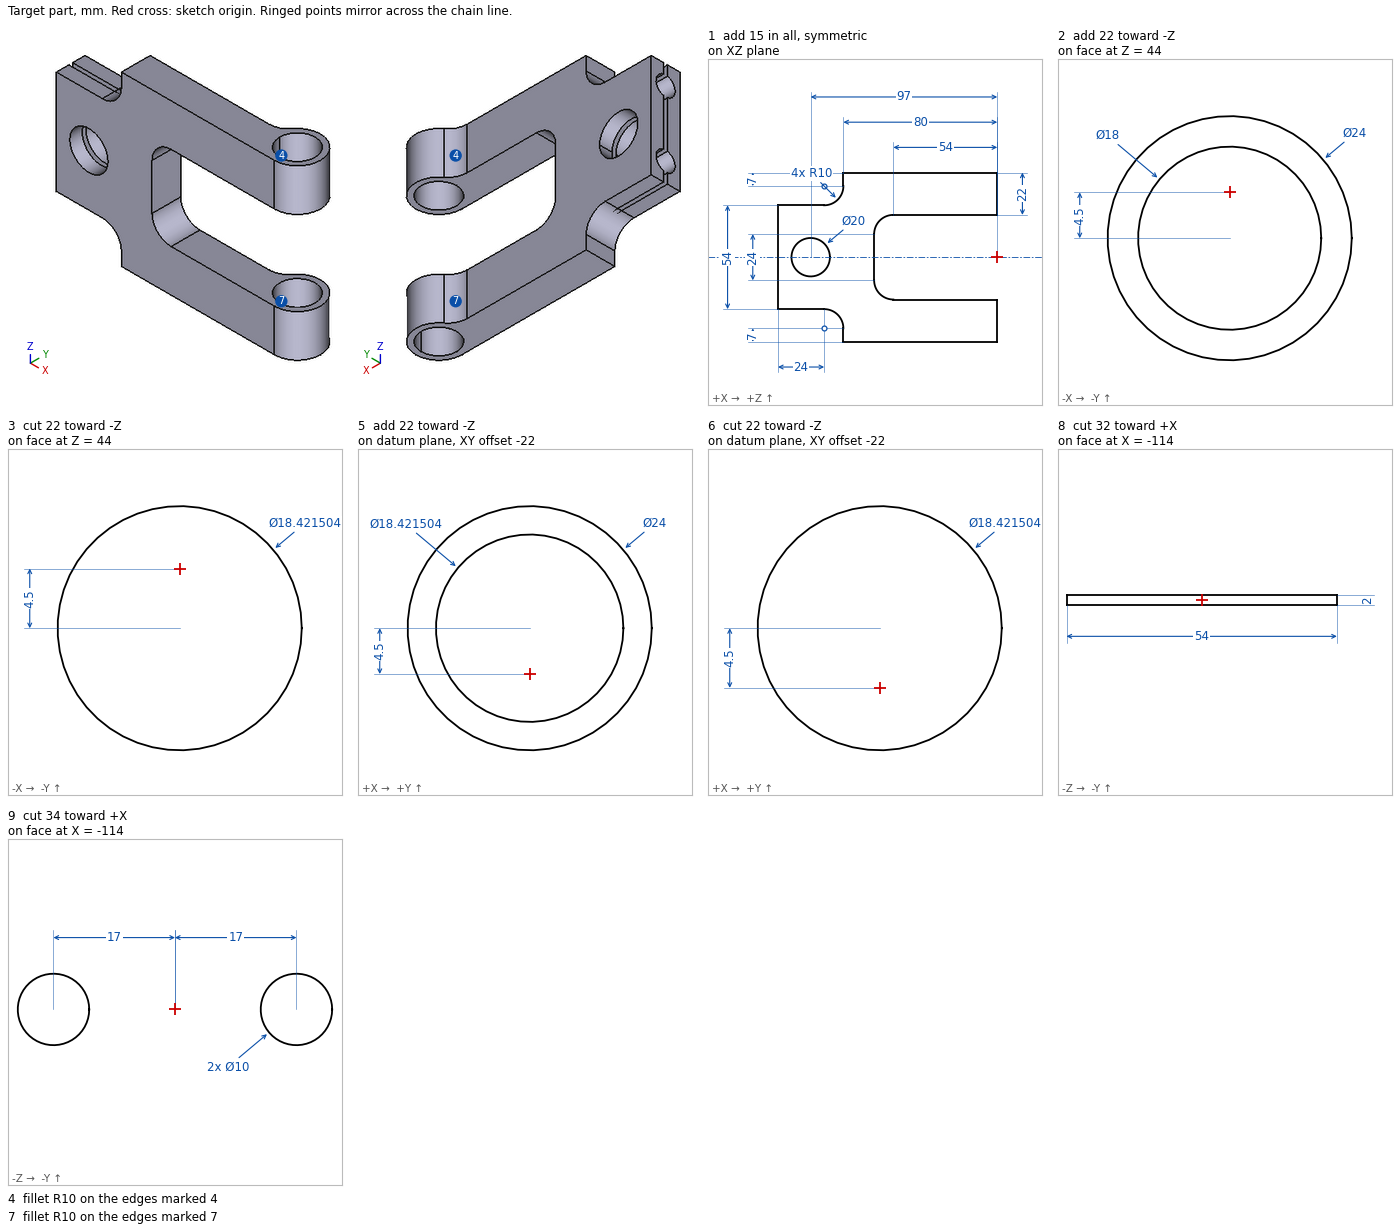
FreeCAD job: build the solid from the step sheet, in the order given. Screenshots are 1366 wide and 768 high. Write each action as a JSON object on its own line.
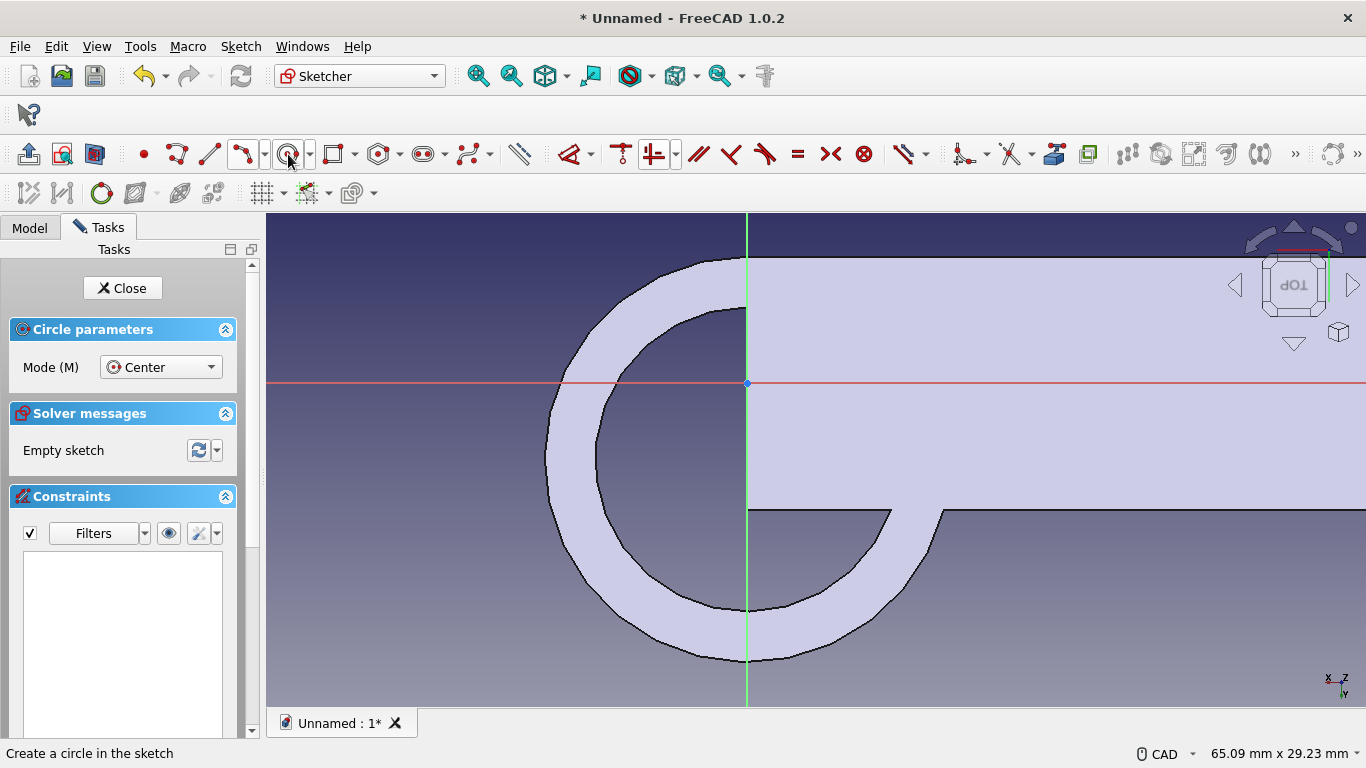
{"action": "left_click", "coordinate": [747, 459]}
{"action": "left_click", "coordinate": [857, 349]}
{"action": "key", "text": "Escape"}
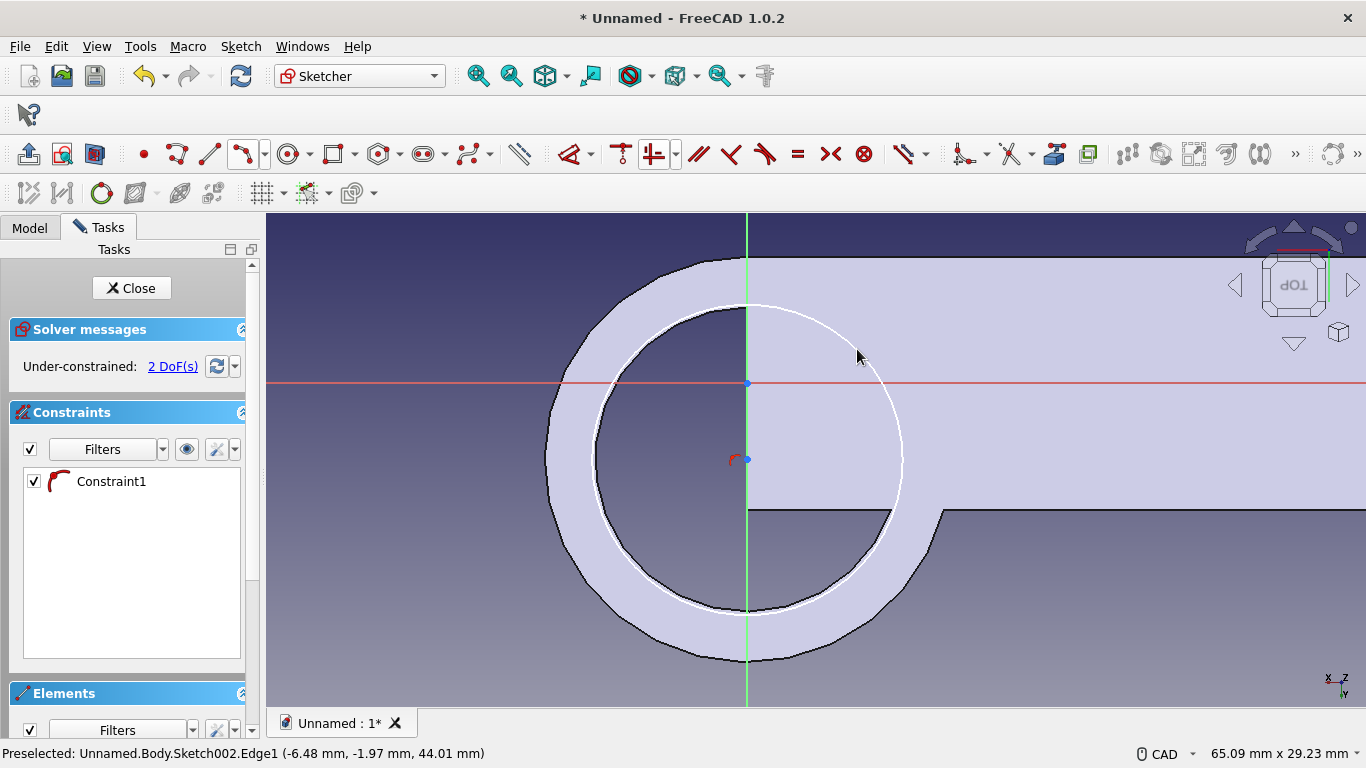
{"action": "left_click", "coordinate": [568, 154]}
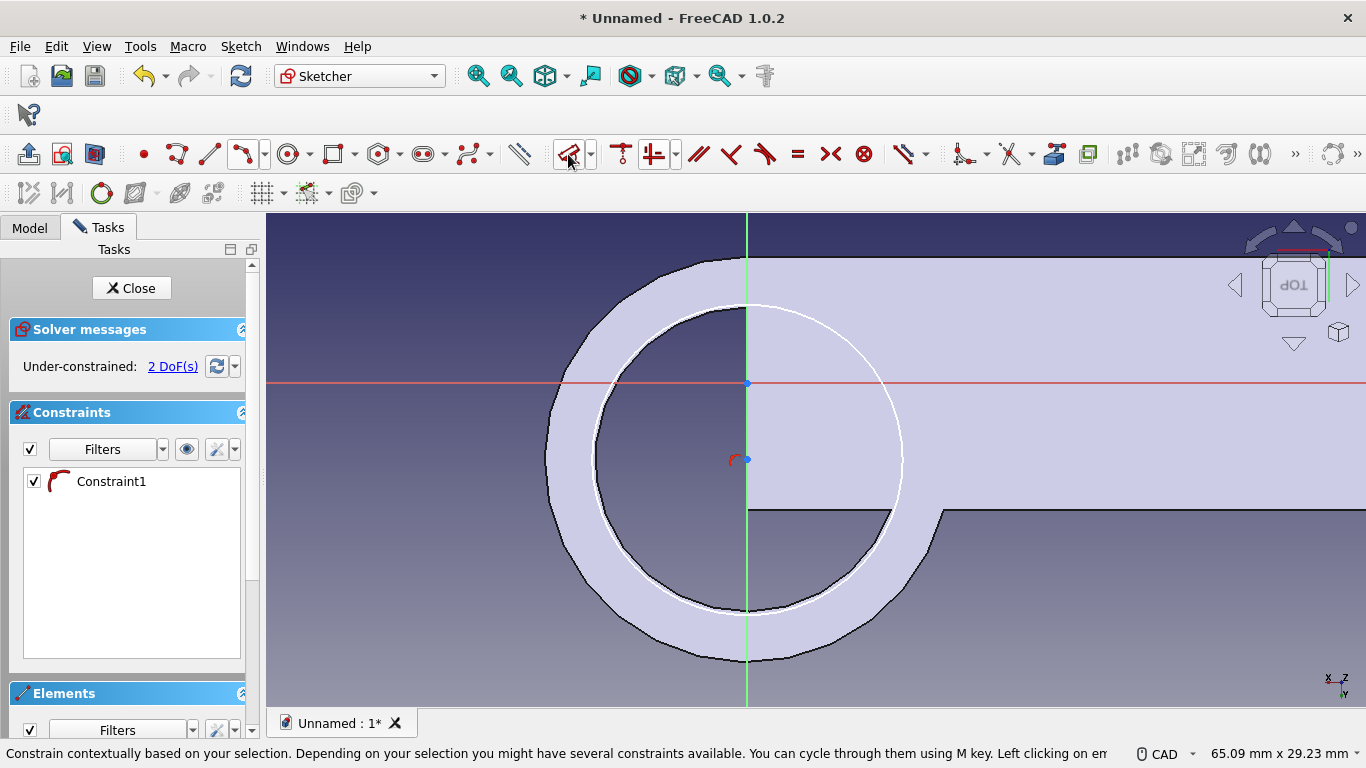
{"action": "left_click", "coordinate": [857, 350]}
{"action": "left_click", "coordinate": [880, 327]}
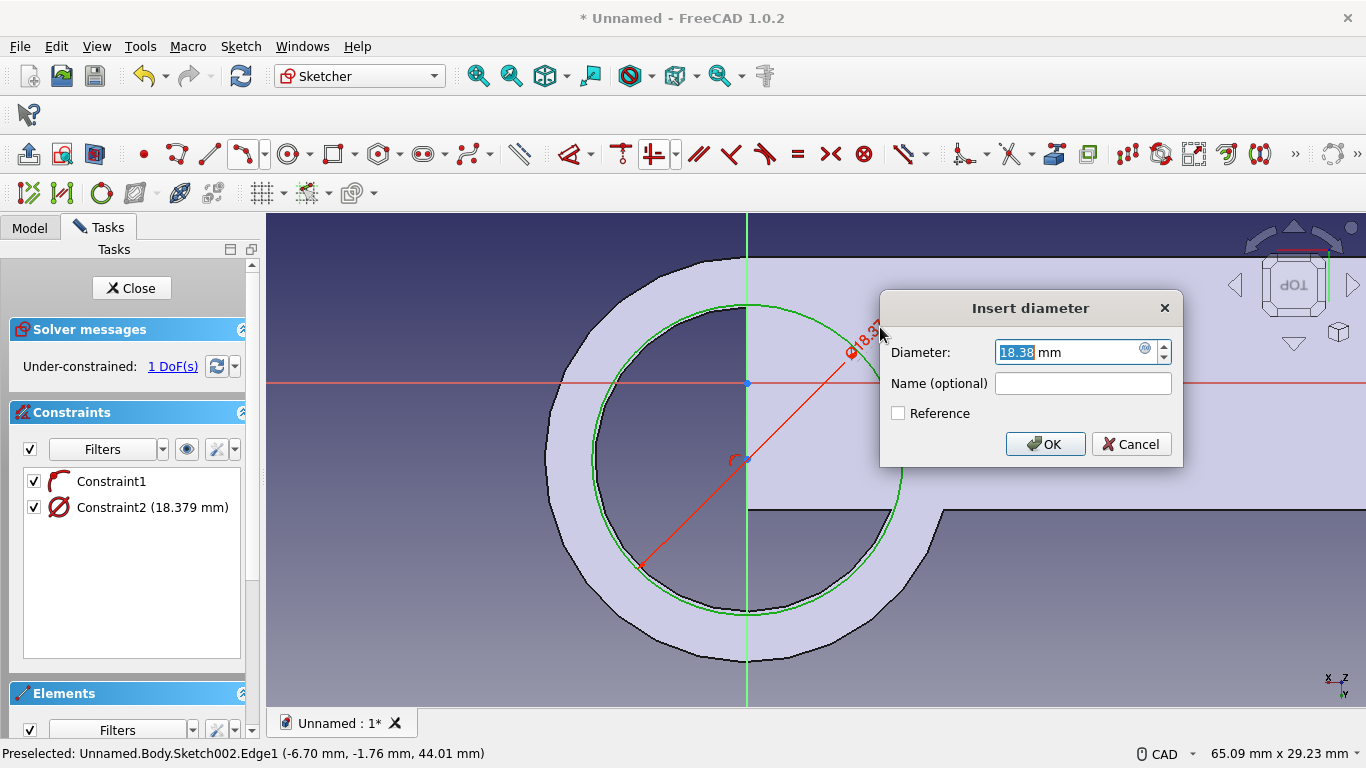
{"action": "type", "text": "18.421504"}
{"action": "key", "text": "Return"}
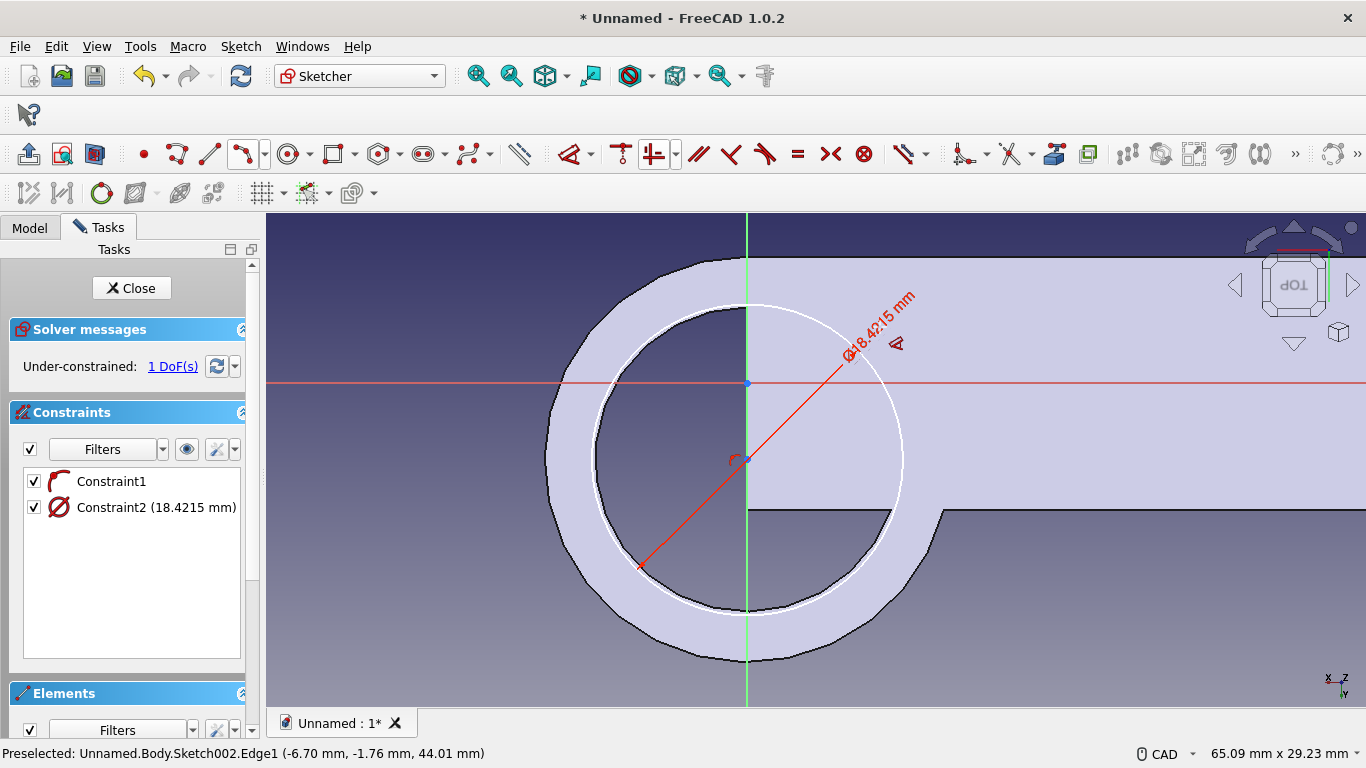
{"action": "left_click", "coordinate": [747, 460]}
{"action": "left_click", "coordinate": [781, 422]}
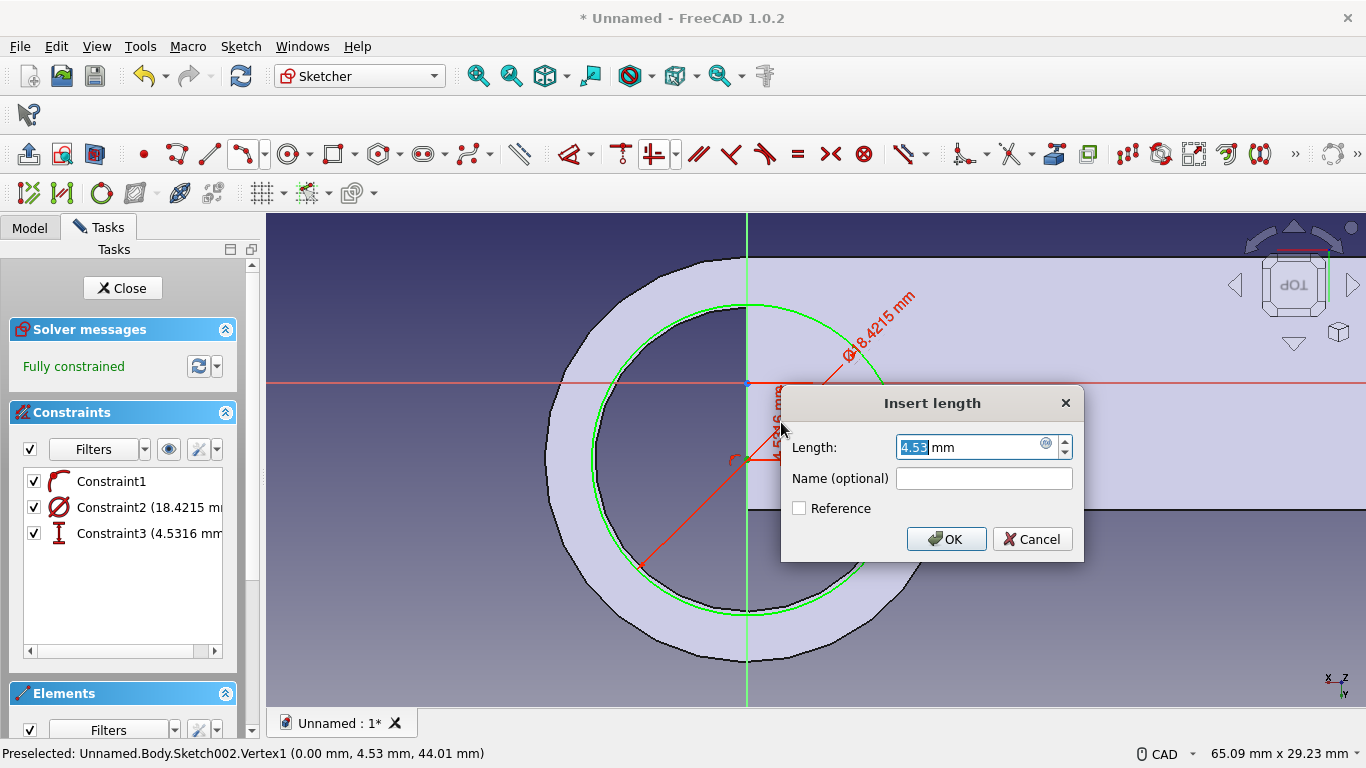
{"action": "type", "text": "4.5"}
{"action": "key", "text": "Return"}
{"action": "key", "text": "Escape"}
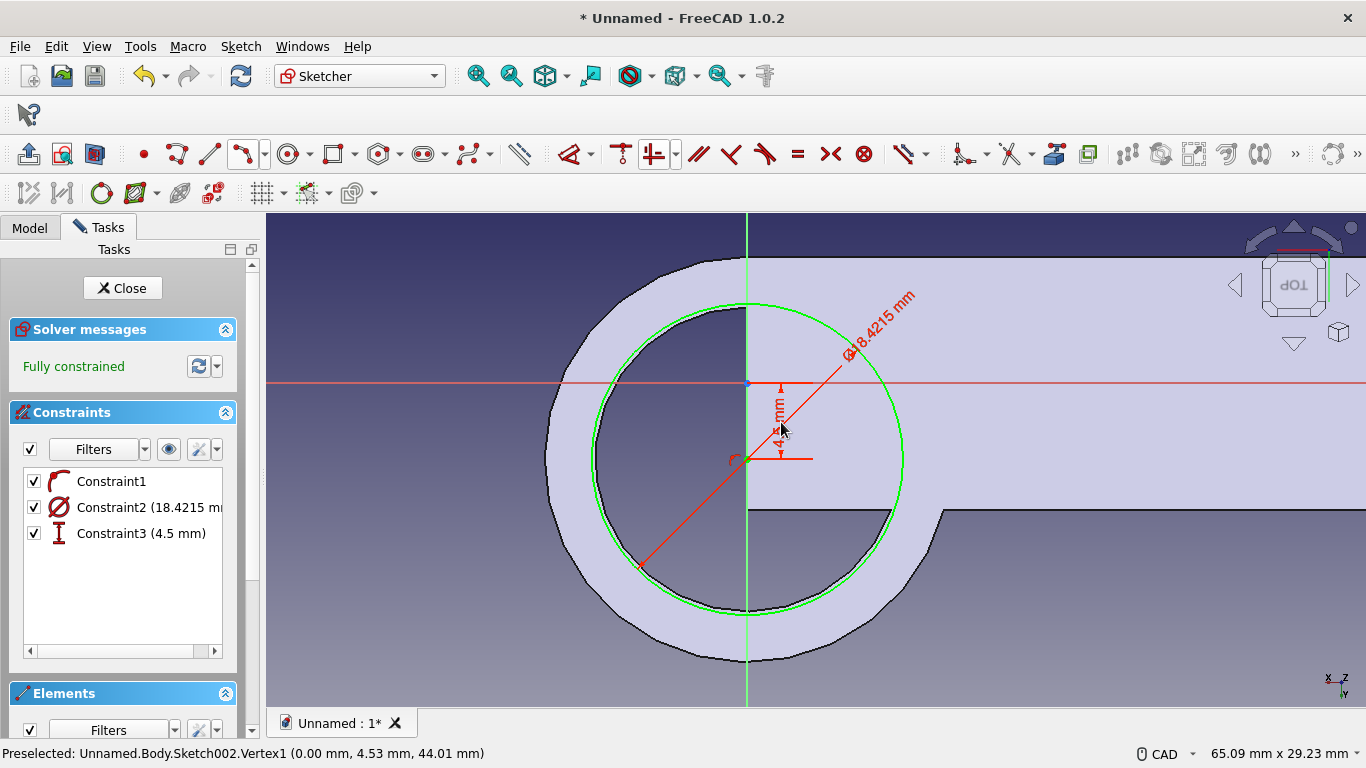
{"action": "left_click", "coordinate": [123, 288]}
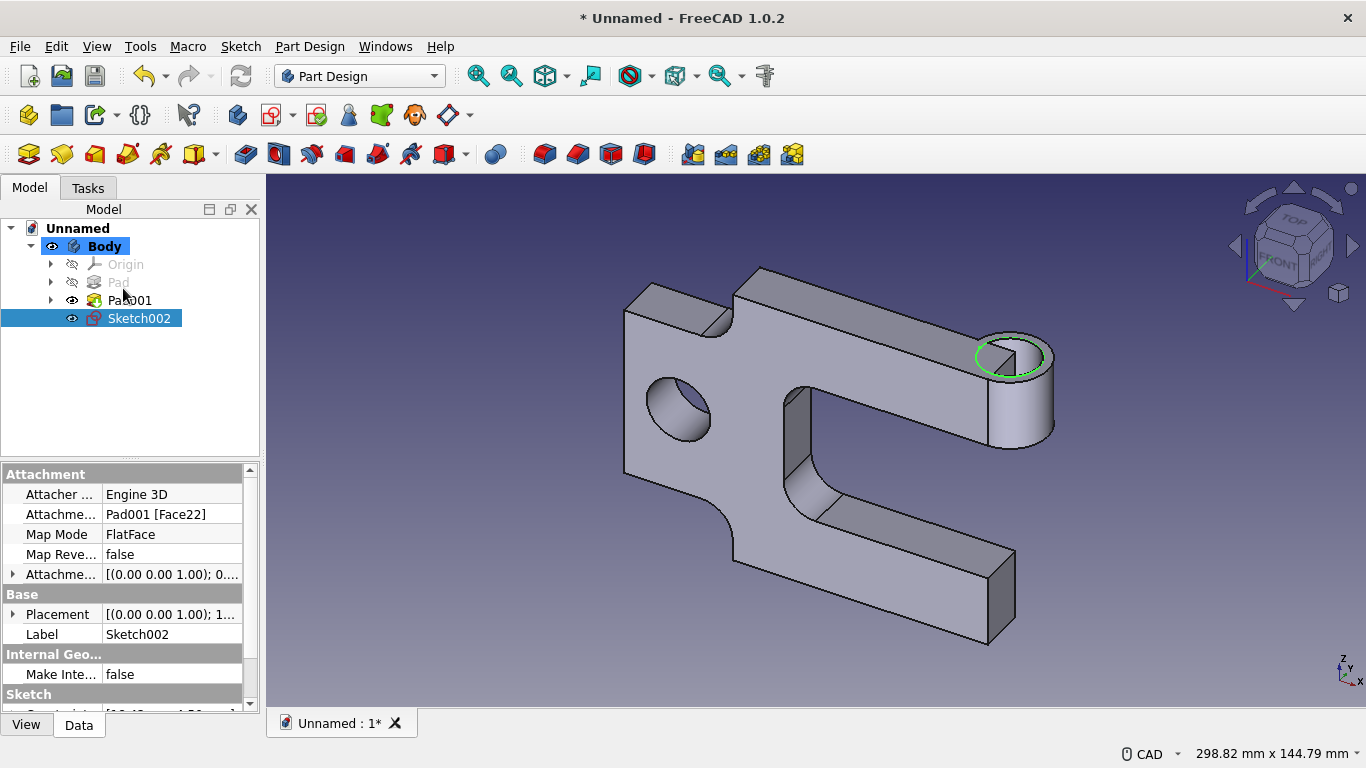
{"action": "left_click", "coordinate": [246, 154]}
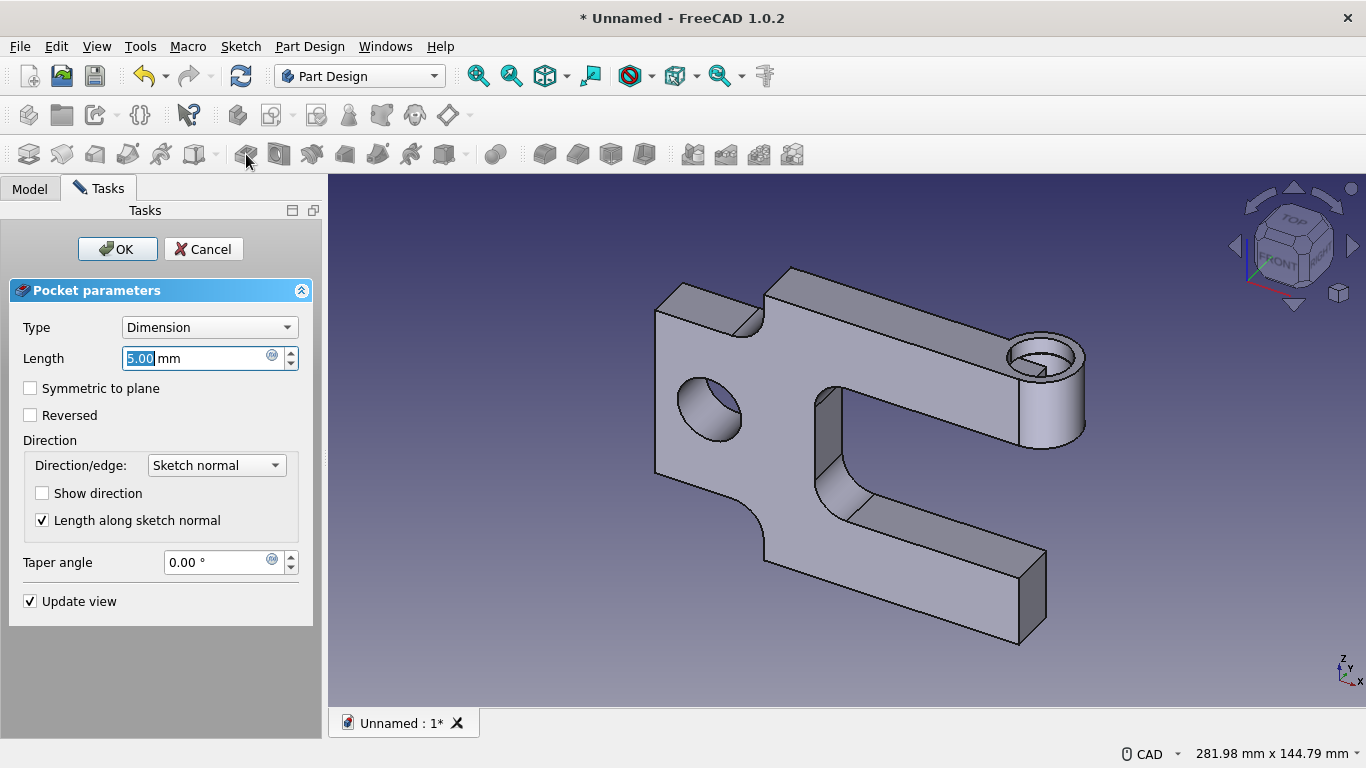
{"action": "type", "text": "22"}
{"action": "key", "text": "Tab"}